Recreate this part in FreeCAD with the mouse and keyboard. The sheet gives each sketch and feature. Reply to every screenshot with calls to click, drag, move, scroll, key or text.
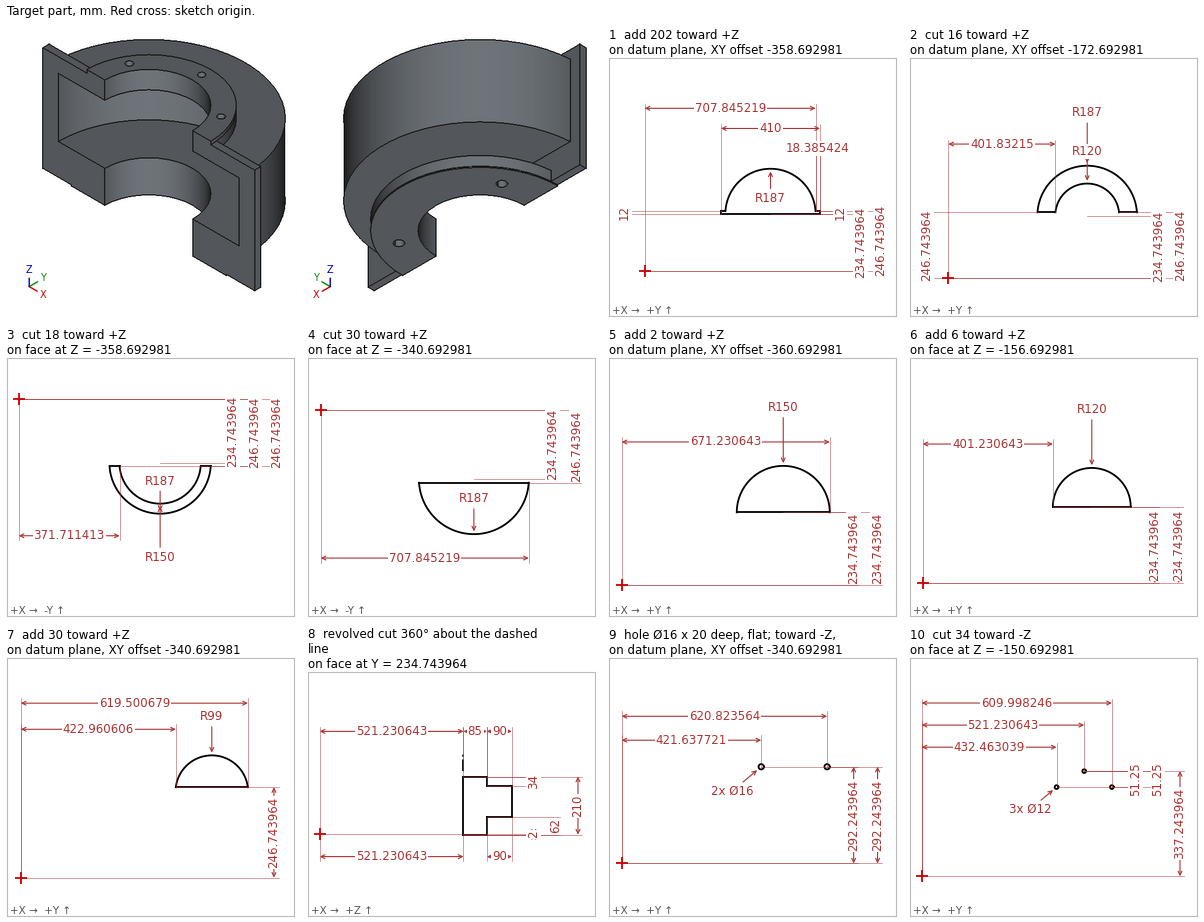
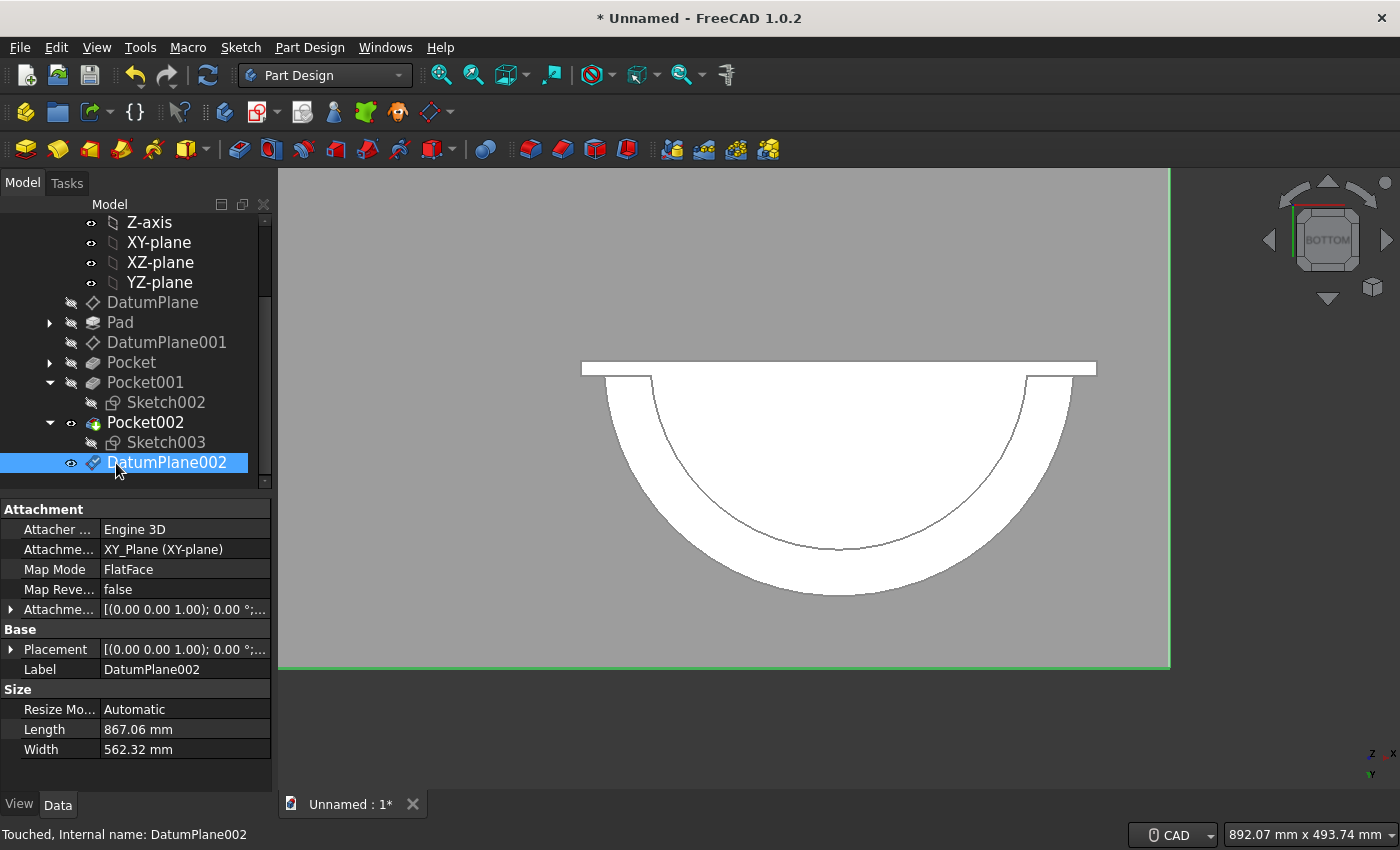
click(258, 112)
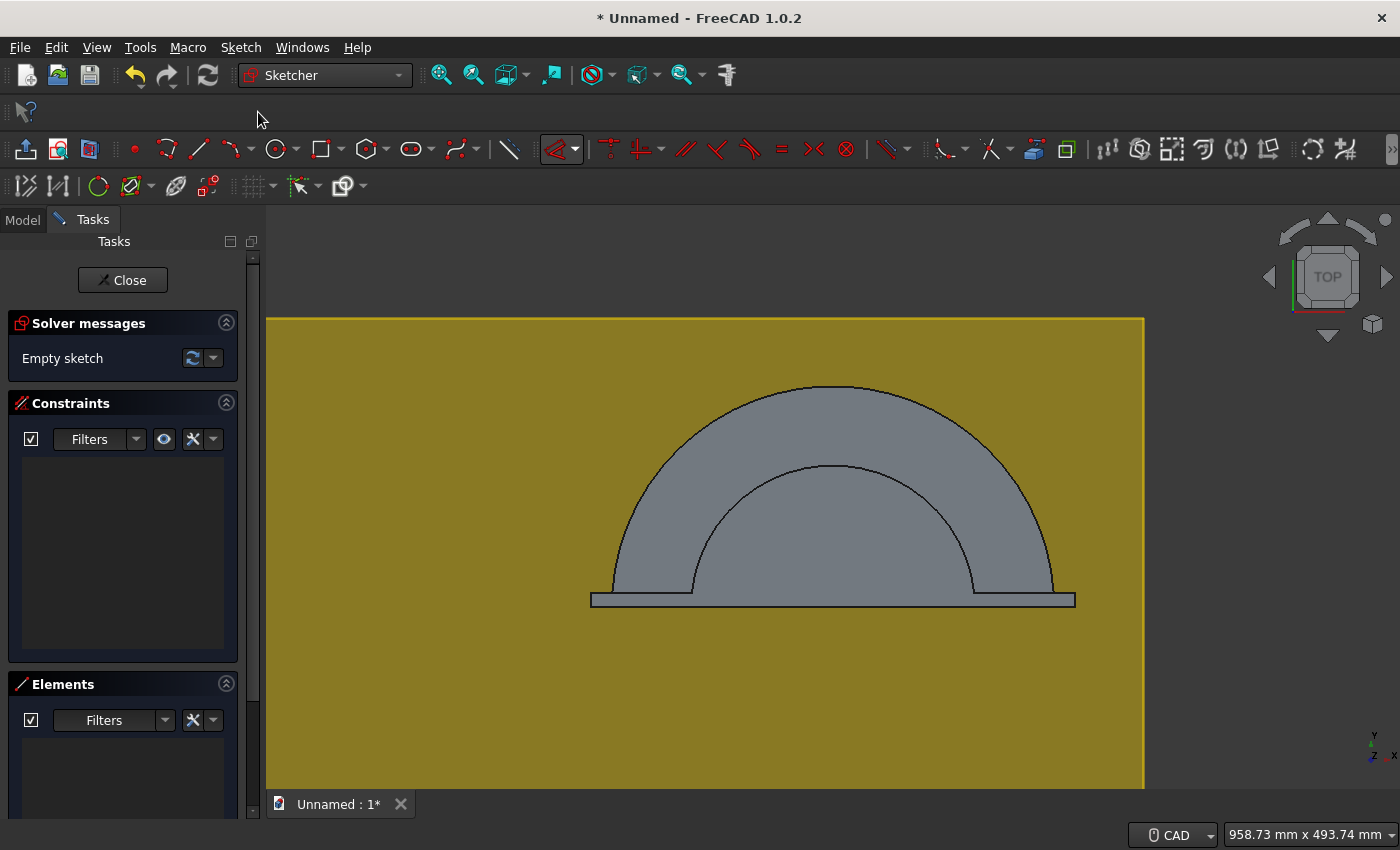
key(q)
key(s)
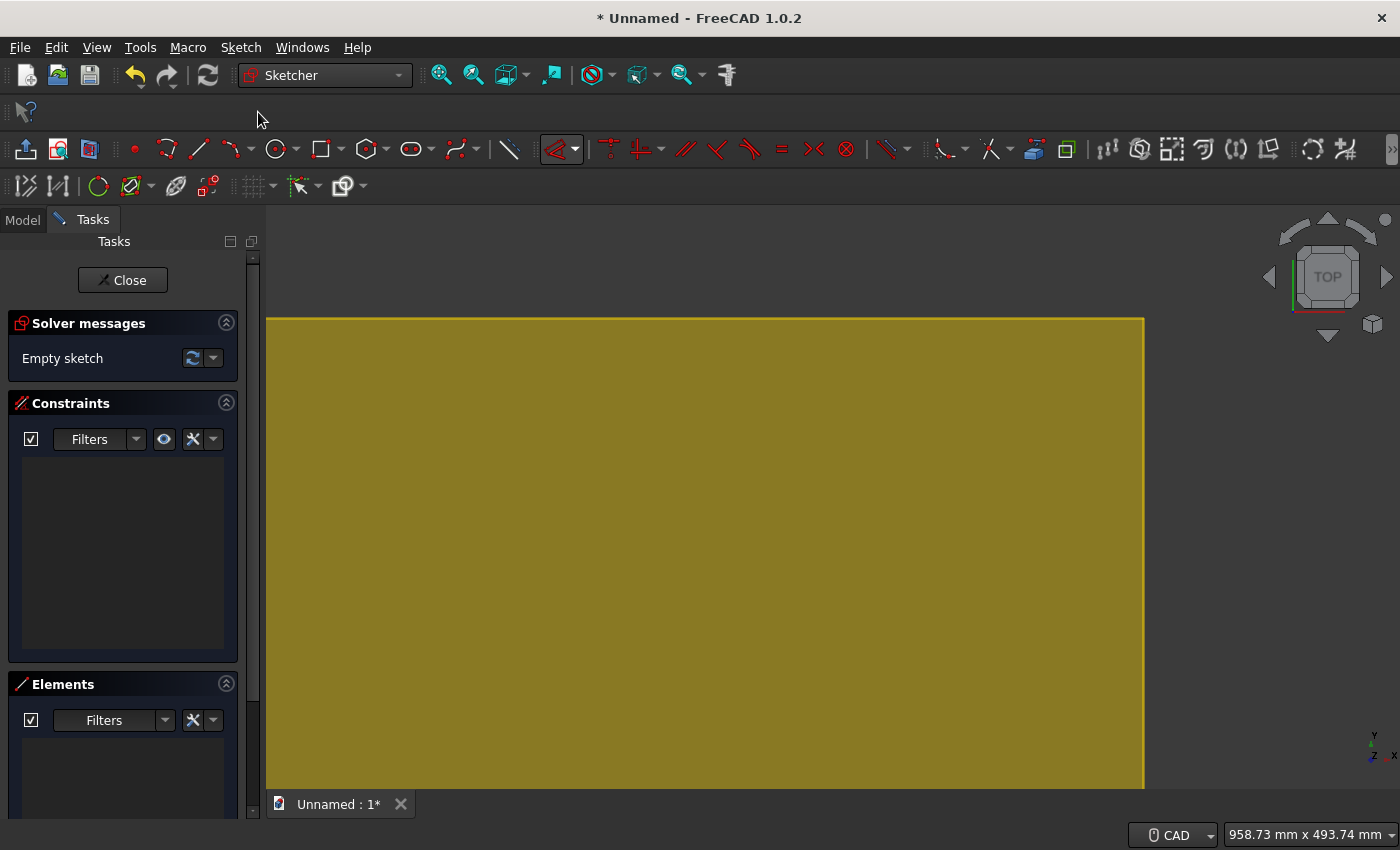
scroll(1072, 233, down, 2)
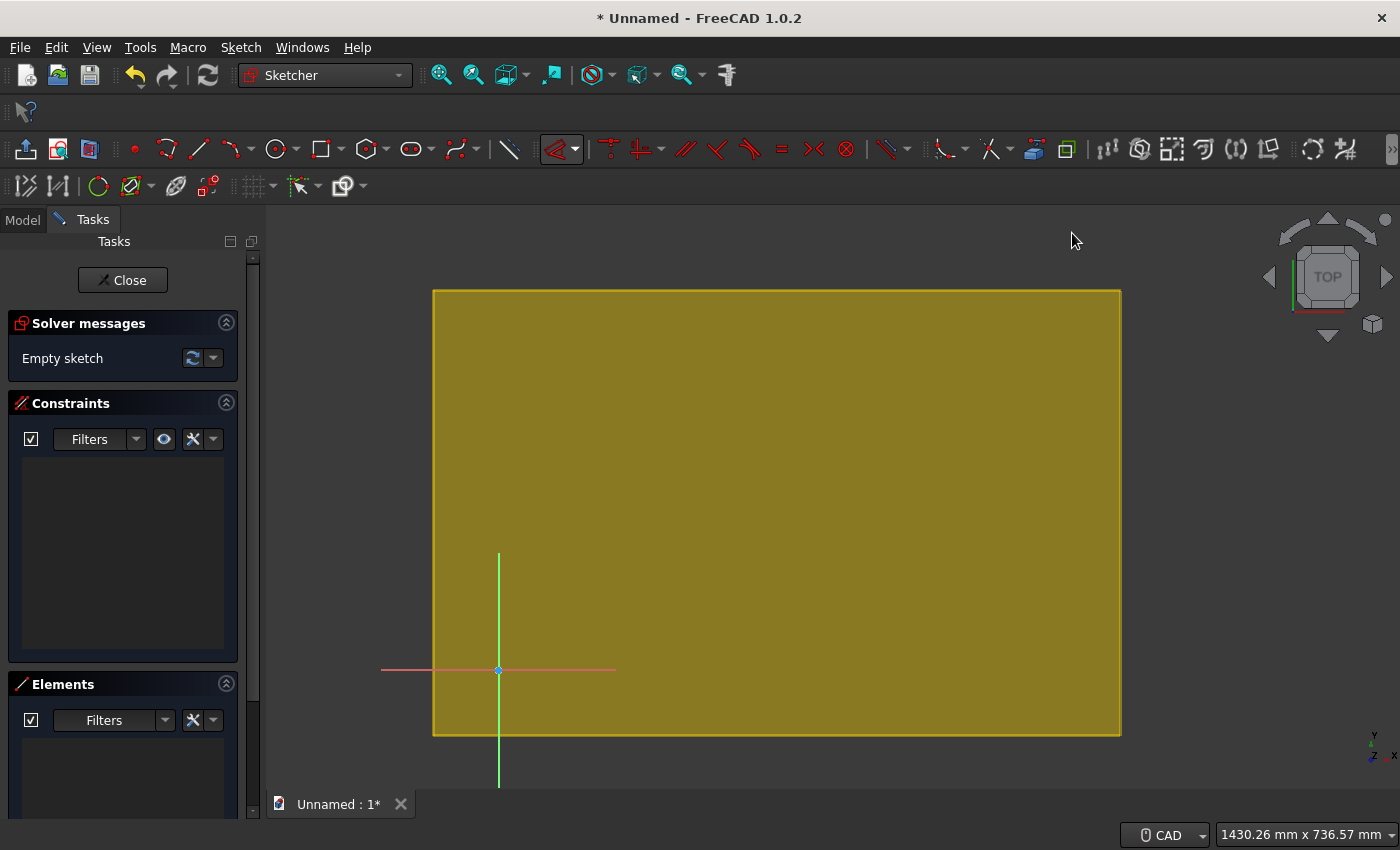
click(200, 150)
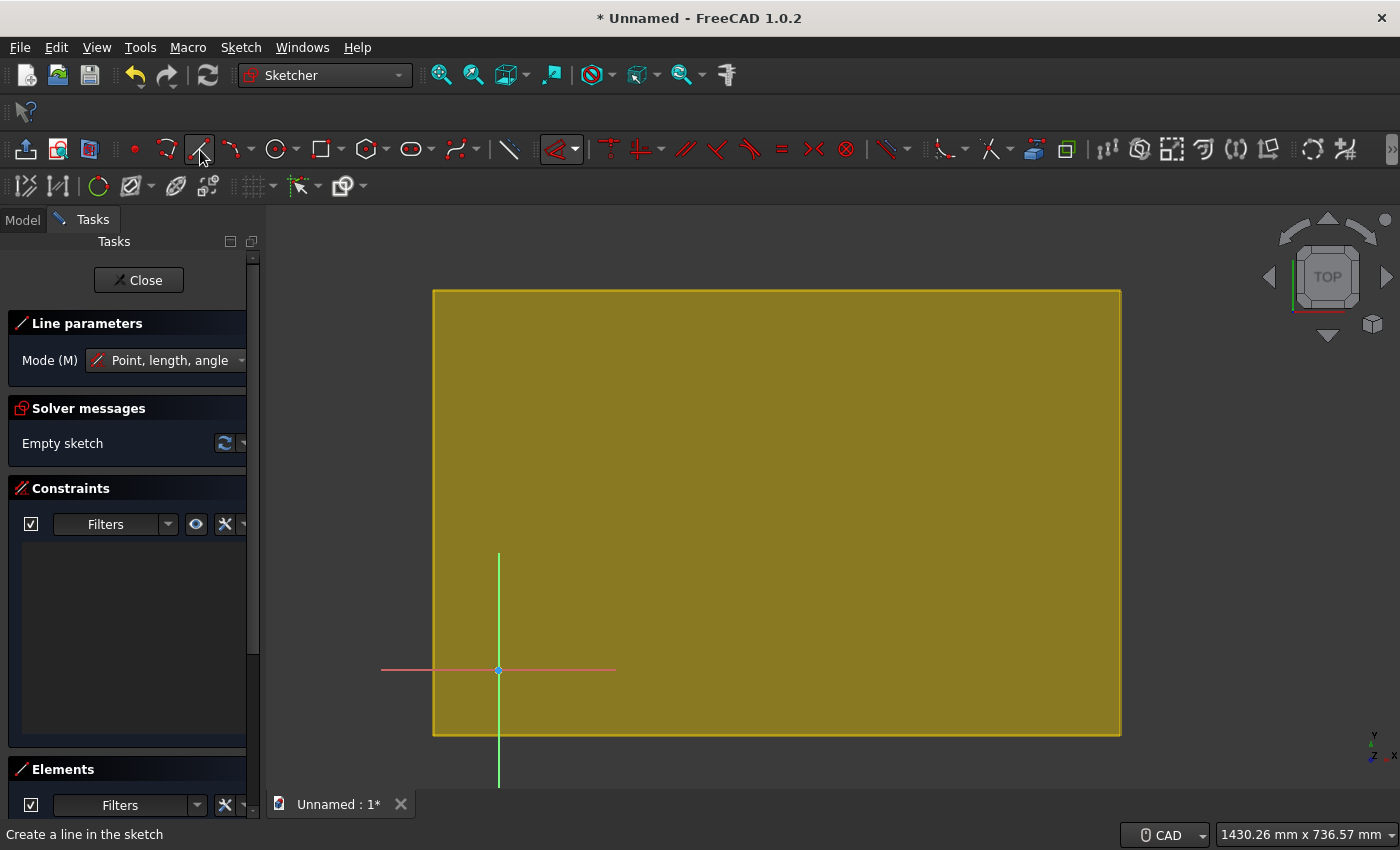
click(1031, 484)
click(793, 484)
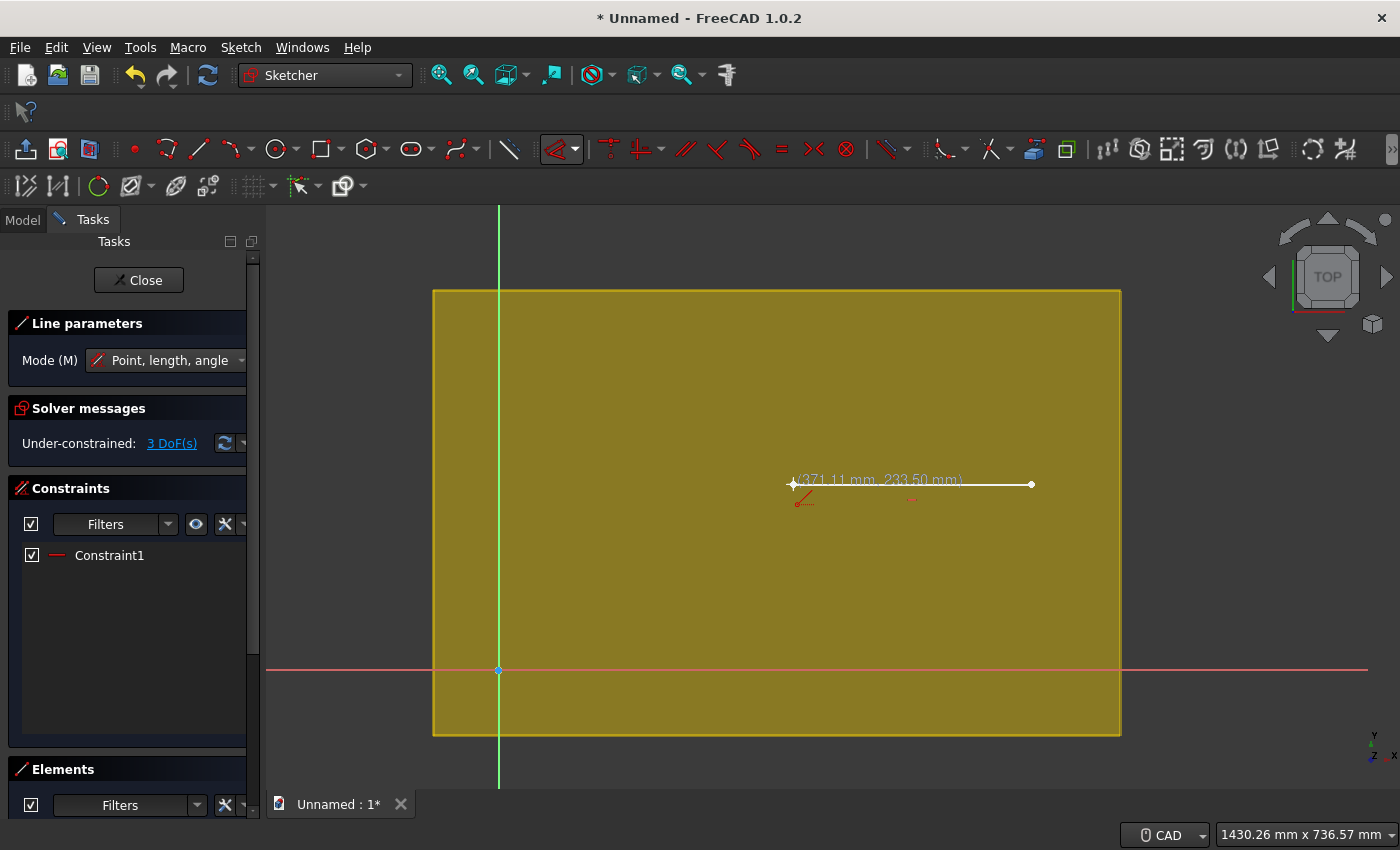
key(g)
key(3)
key(a)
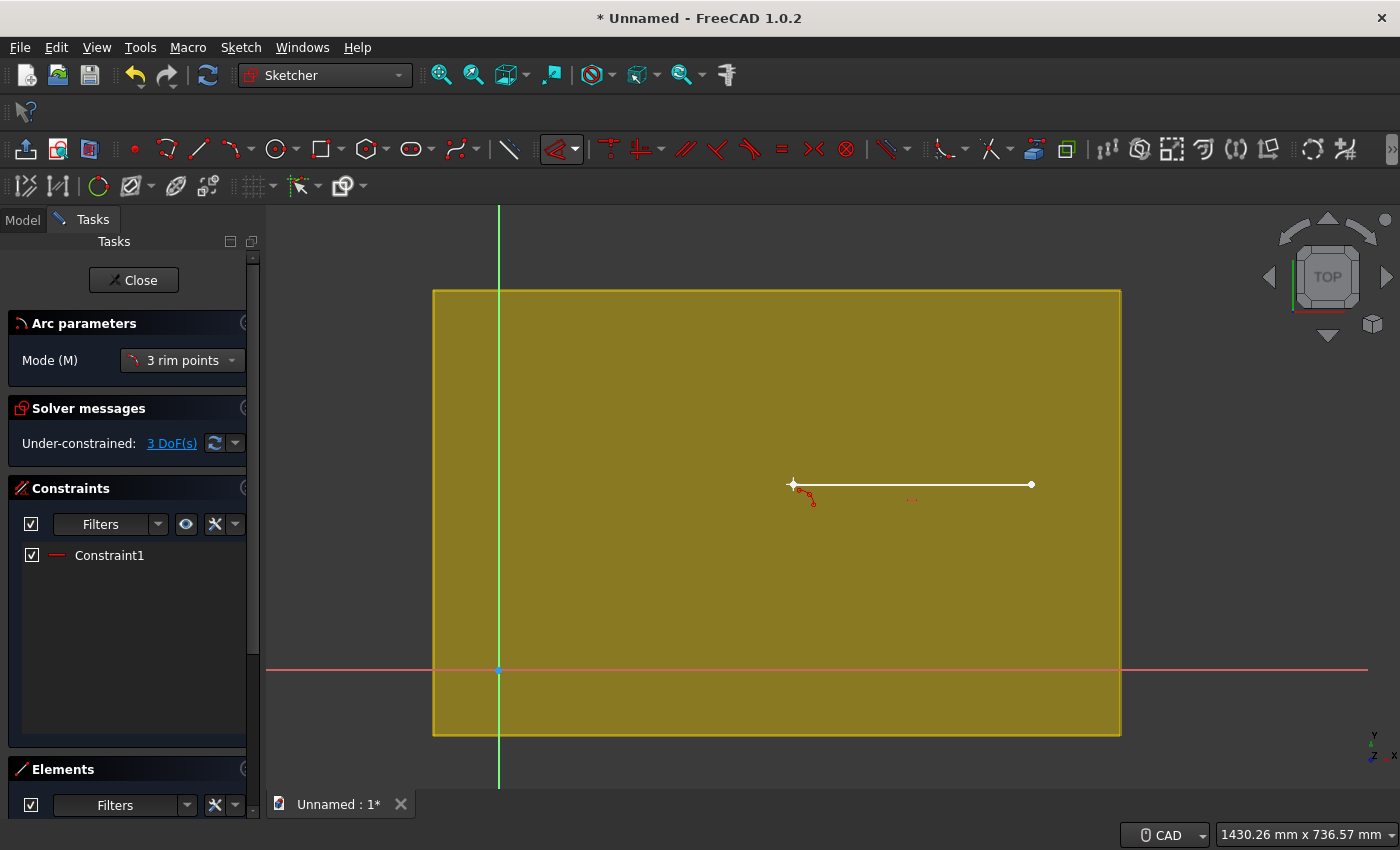
click(793, 485)
click(1031, 485)
click(912, 365)
key(Escape)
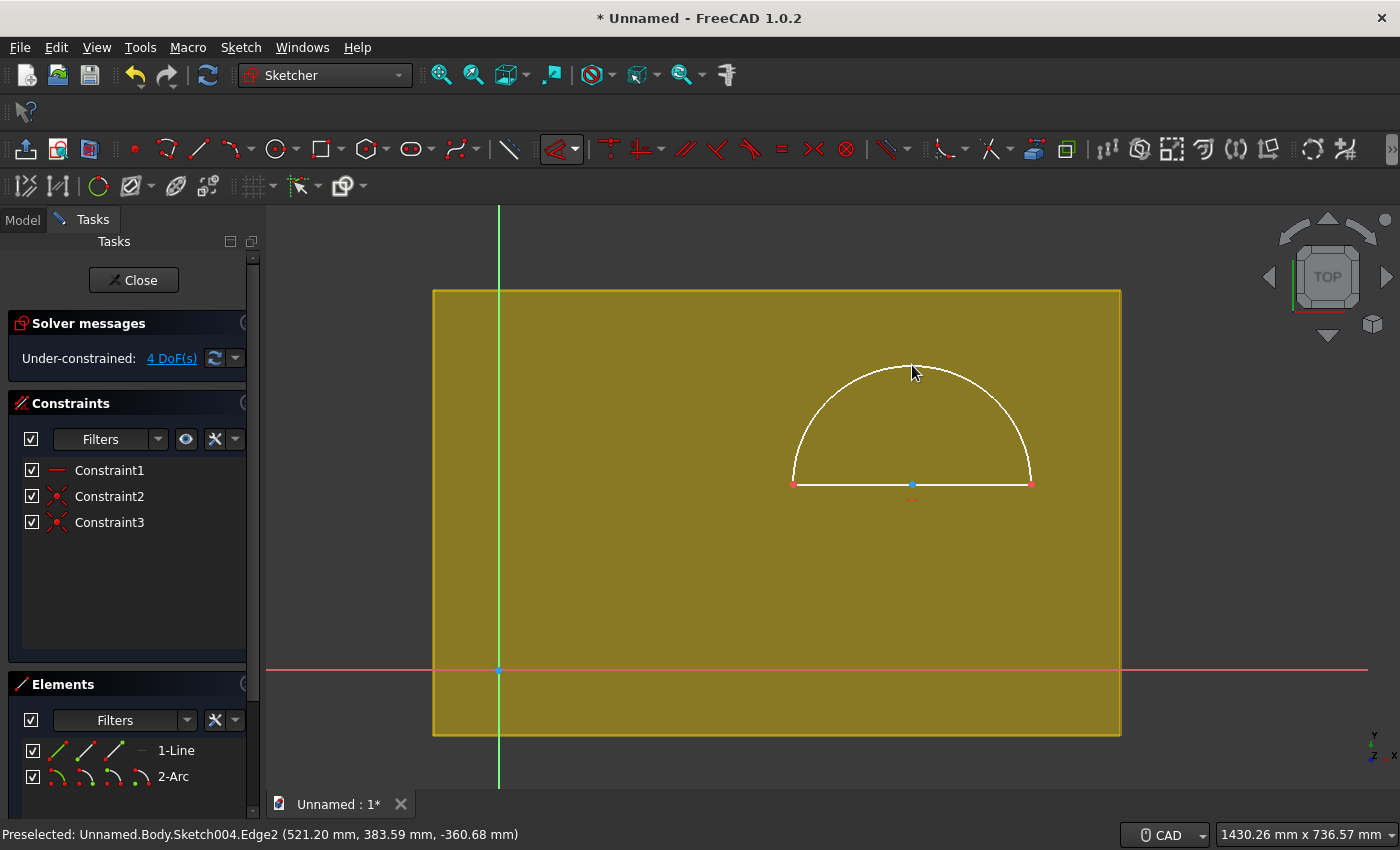
key(d)